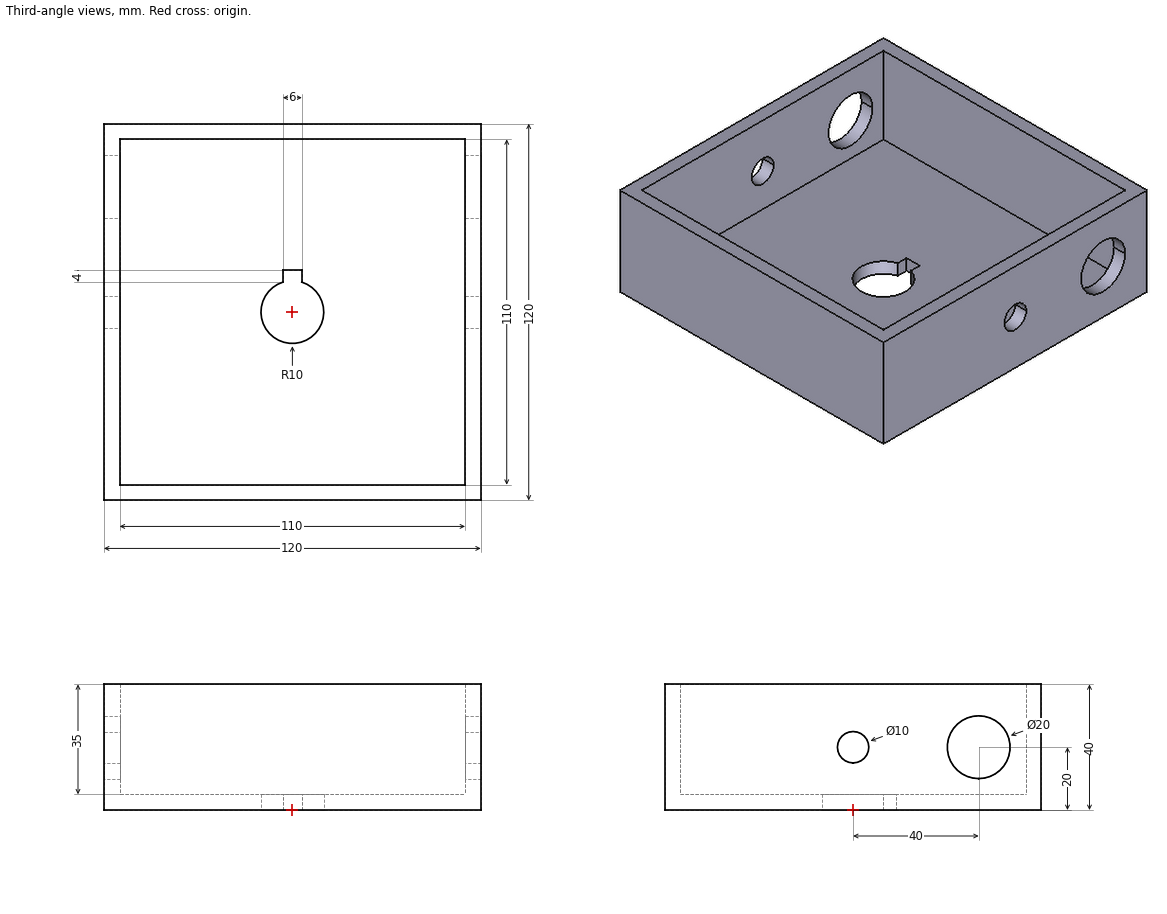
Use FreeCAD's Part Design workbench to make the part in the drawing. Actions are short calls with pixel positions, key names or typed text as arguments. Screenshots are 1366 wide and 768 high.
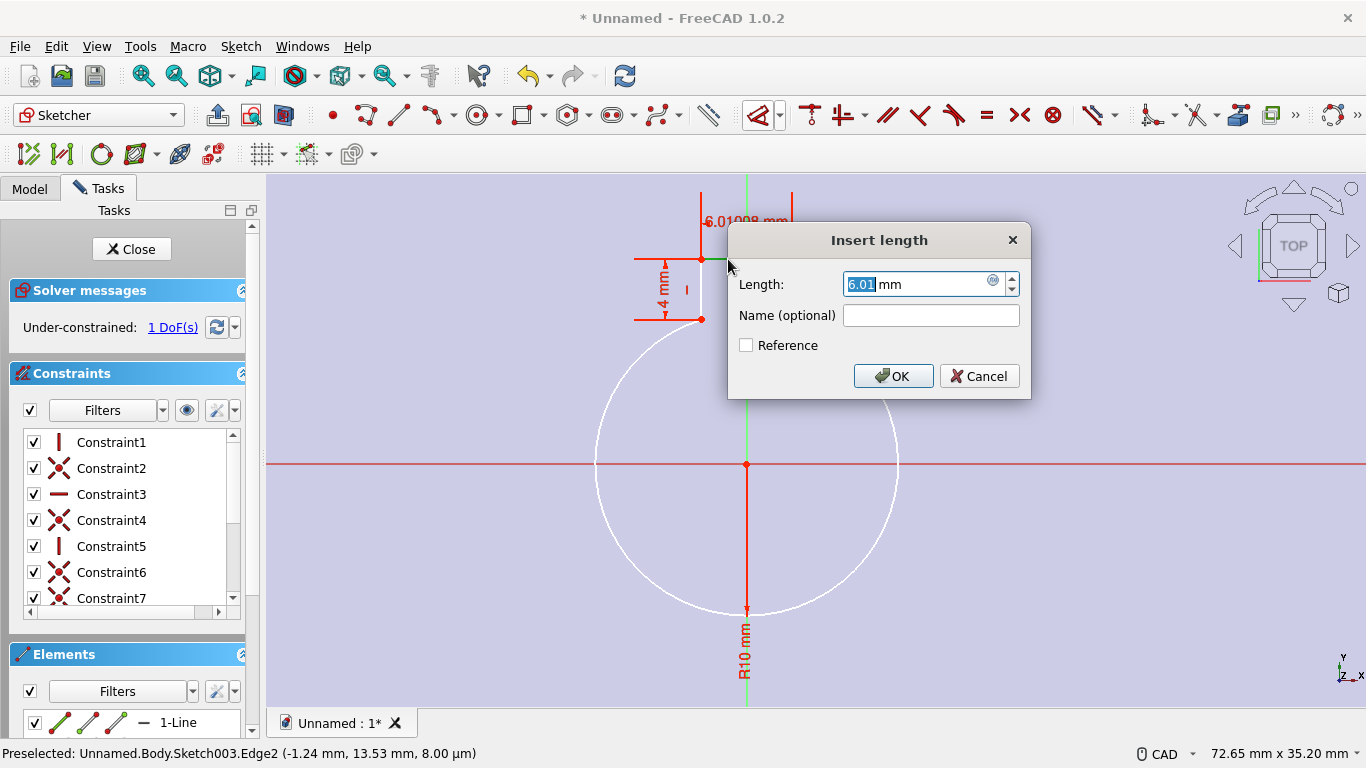
text(6)
key(Return)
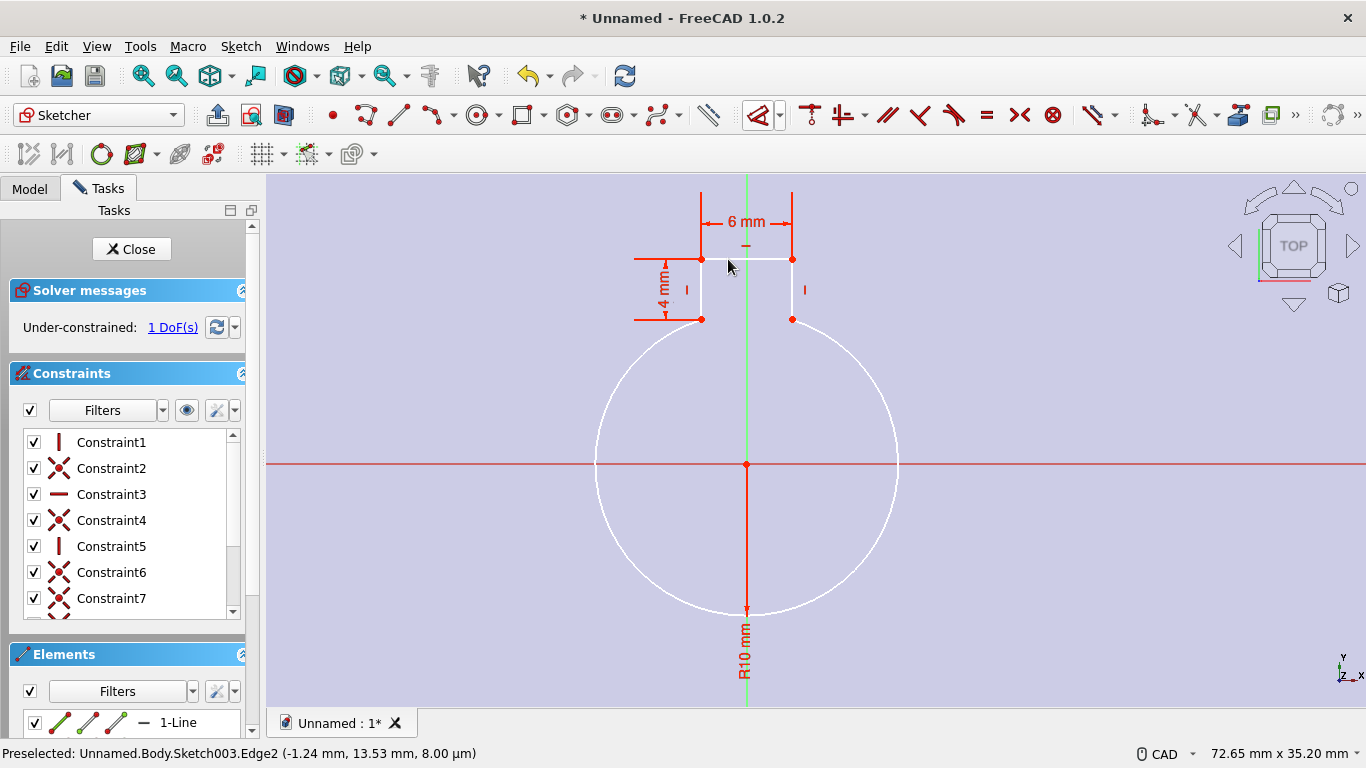
click(792, 277)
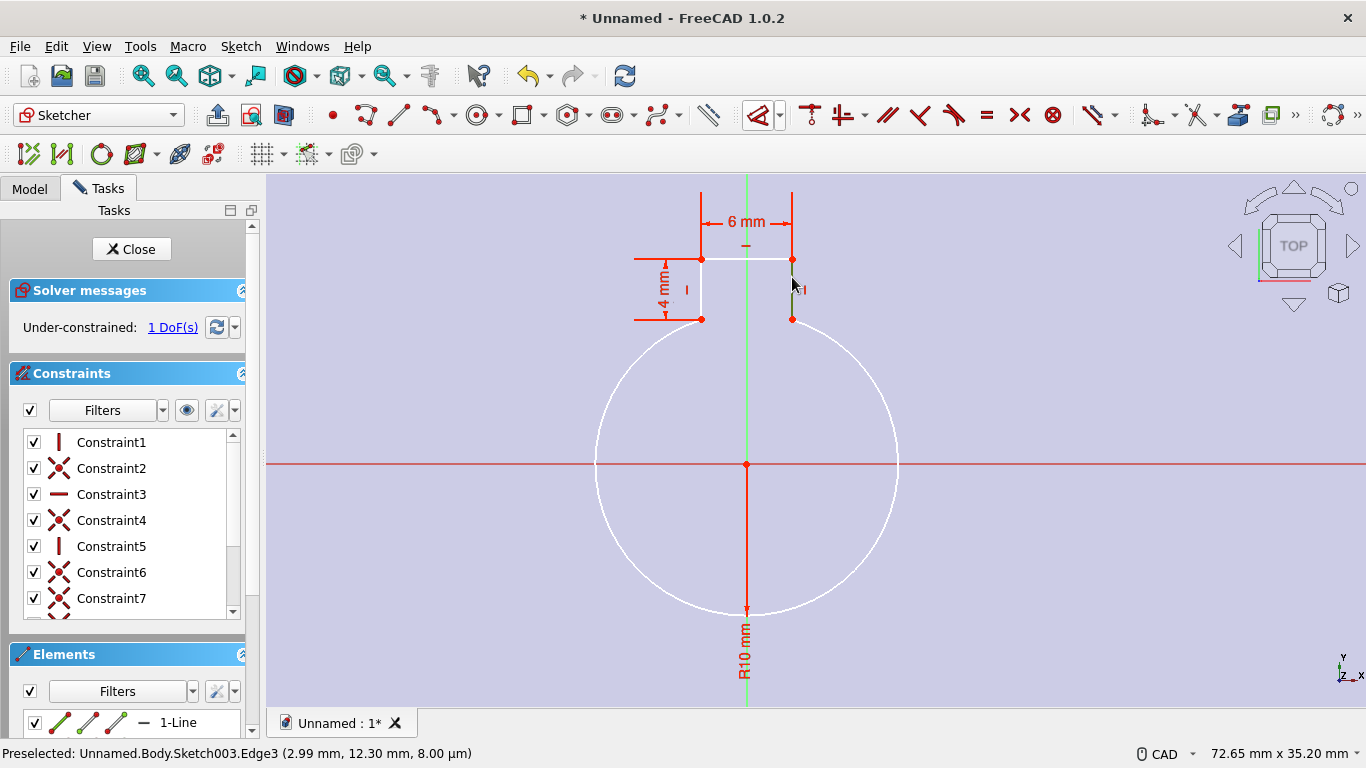
key(i)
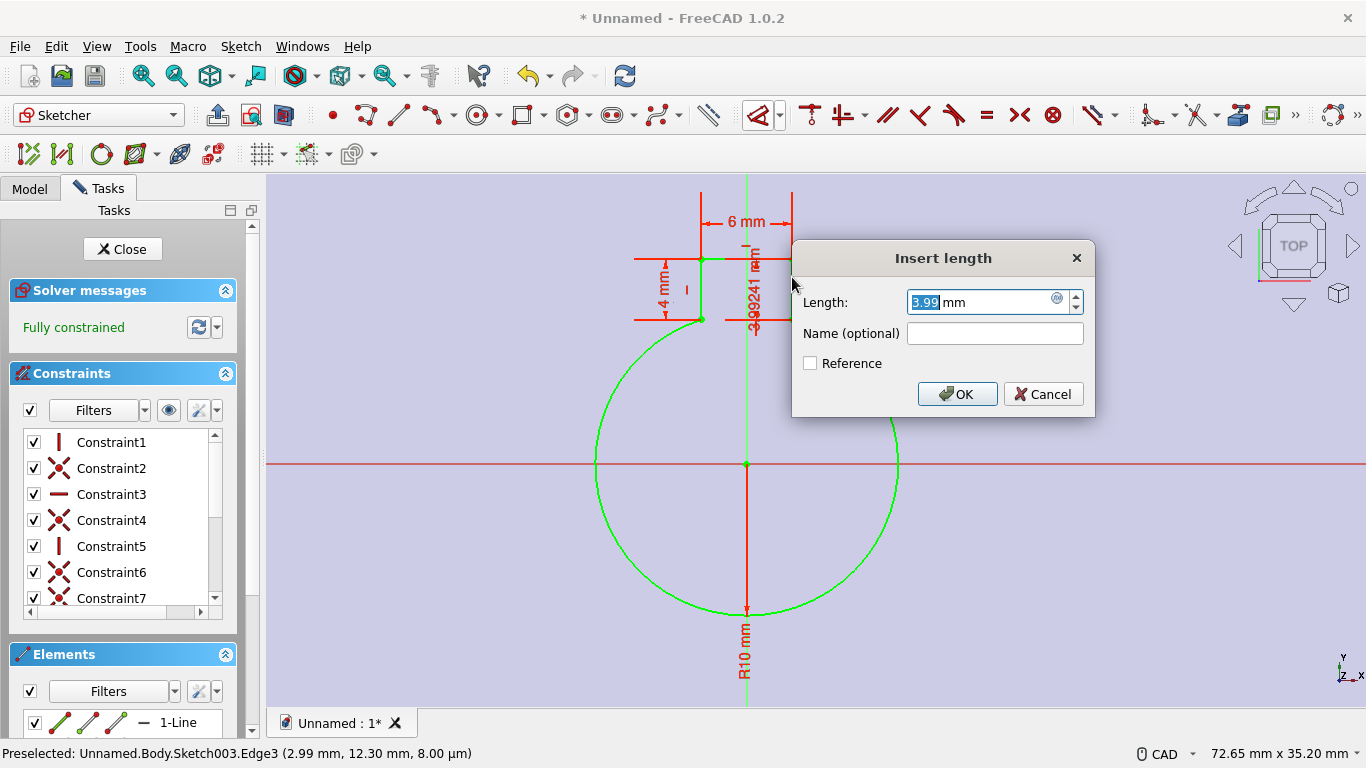
text(4)
key(Return)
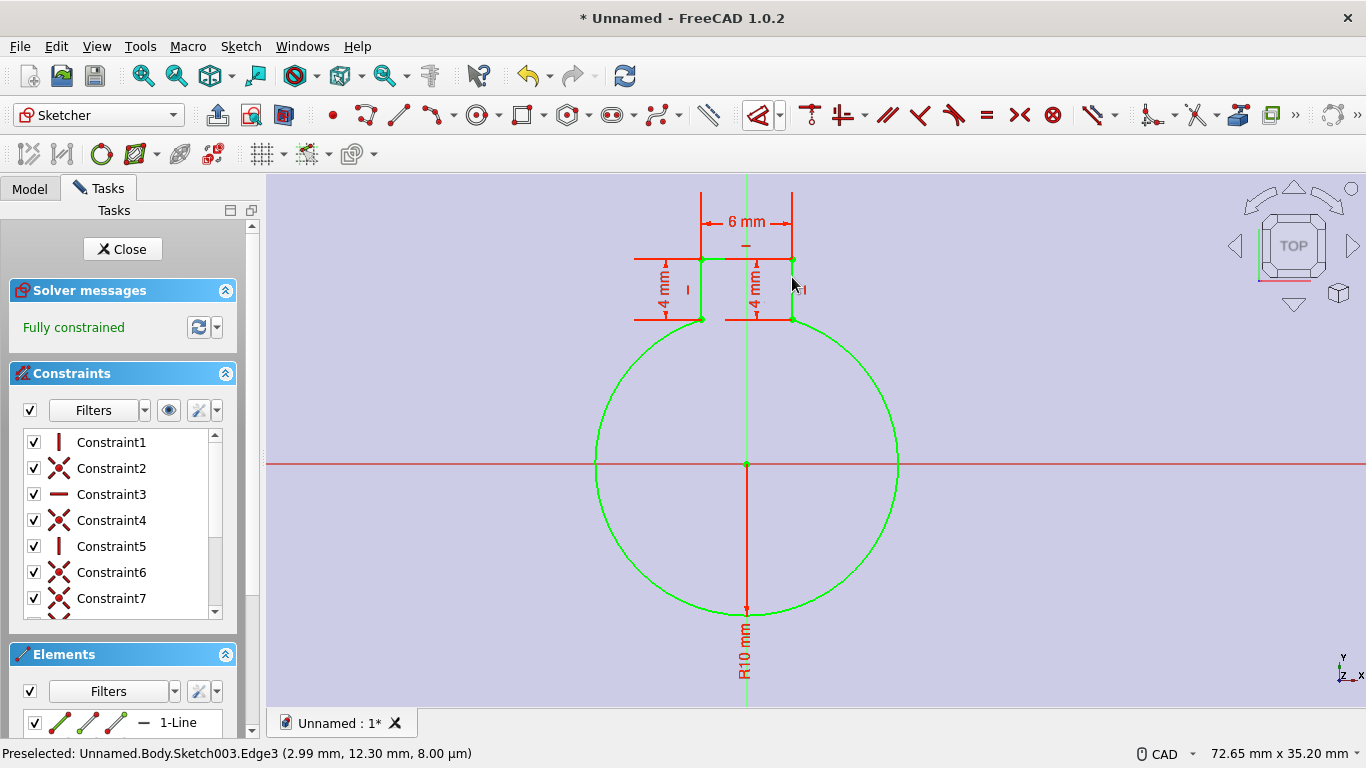
click(123, 249)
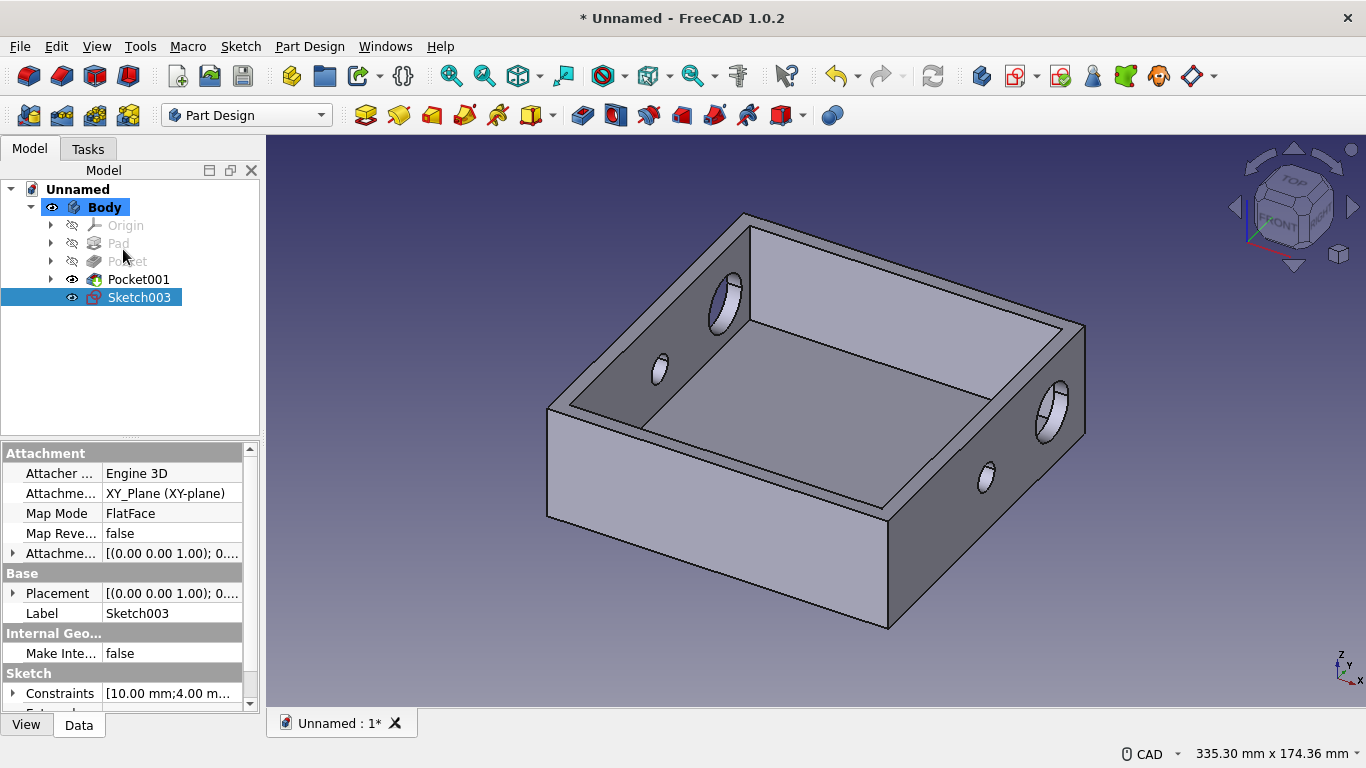
click(583, 116)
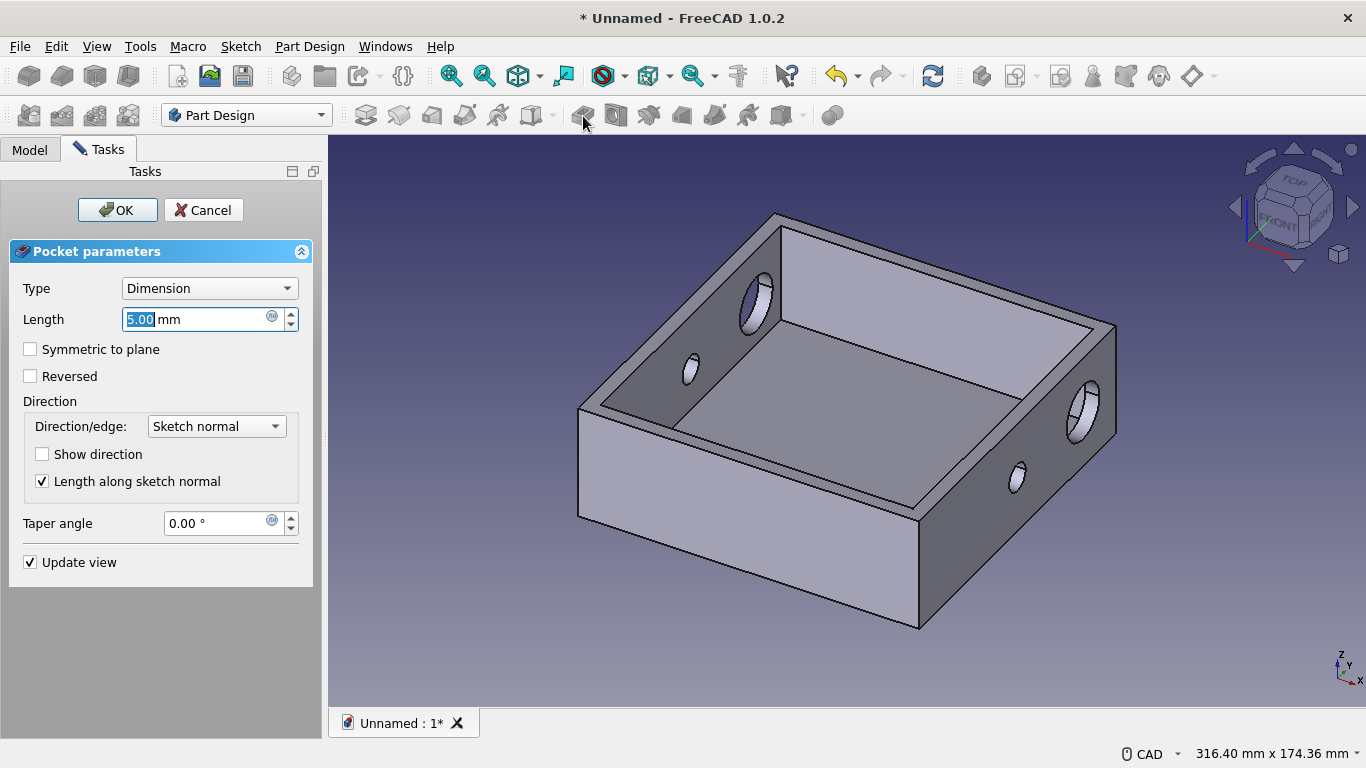
click(210, 288)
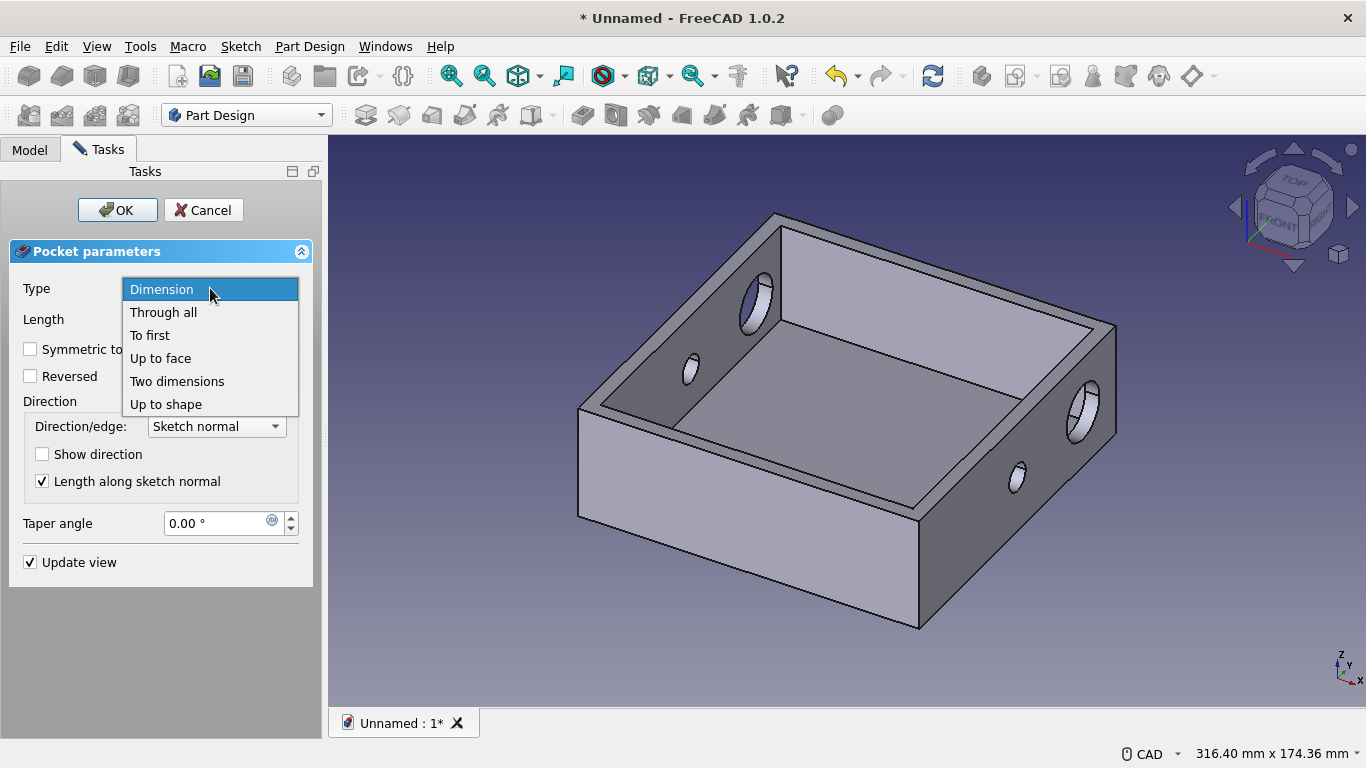
click(208, 312)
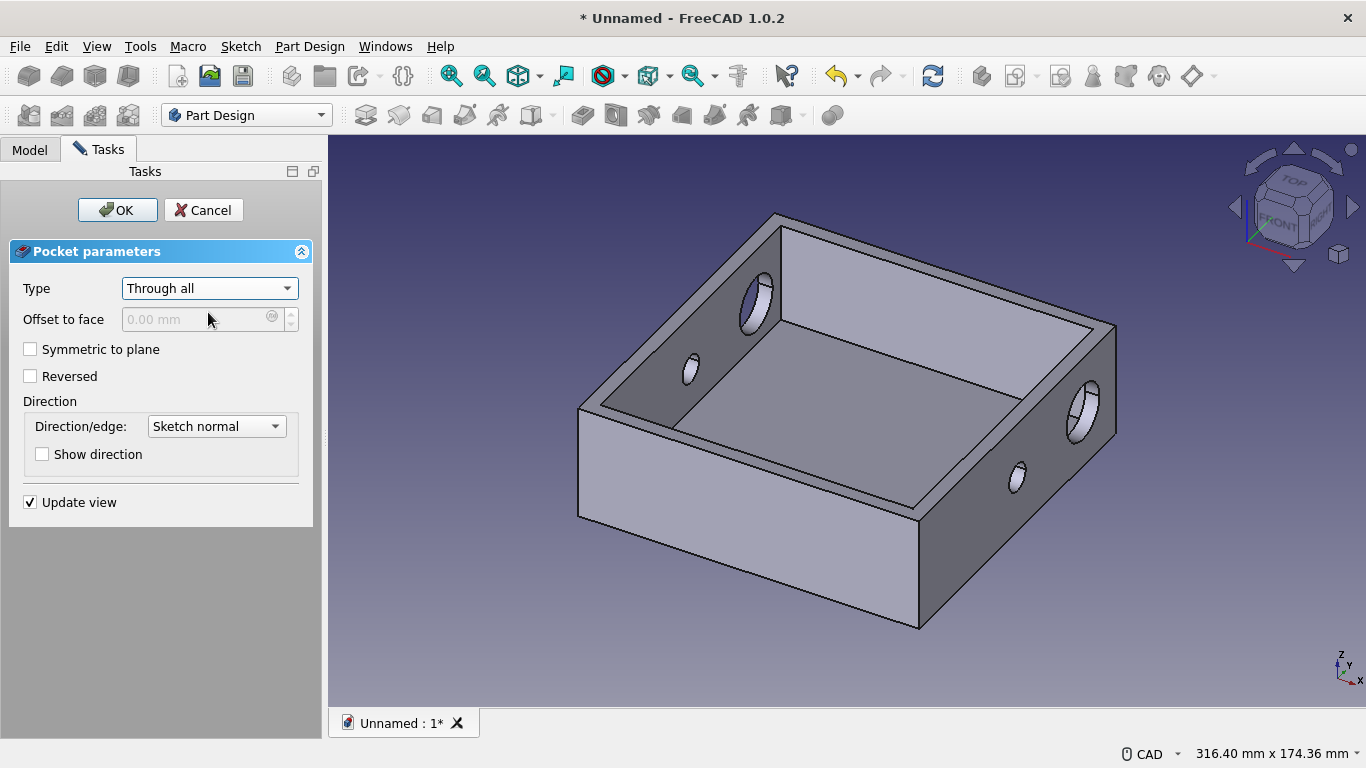
click(31, 376)